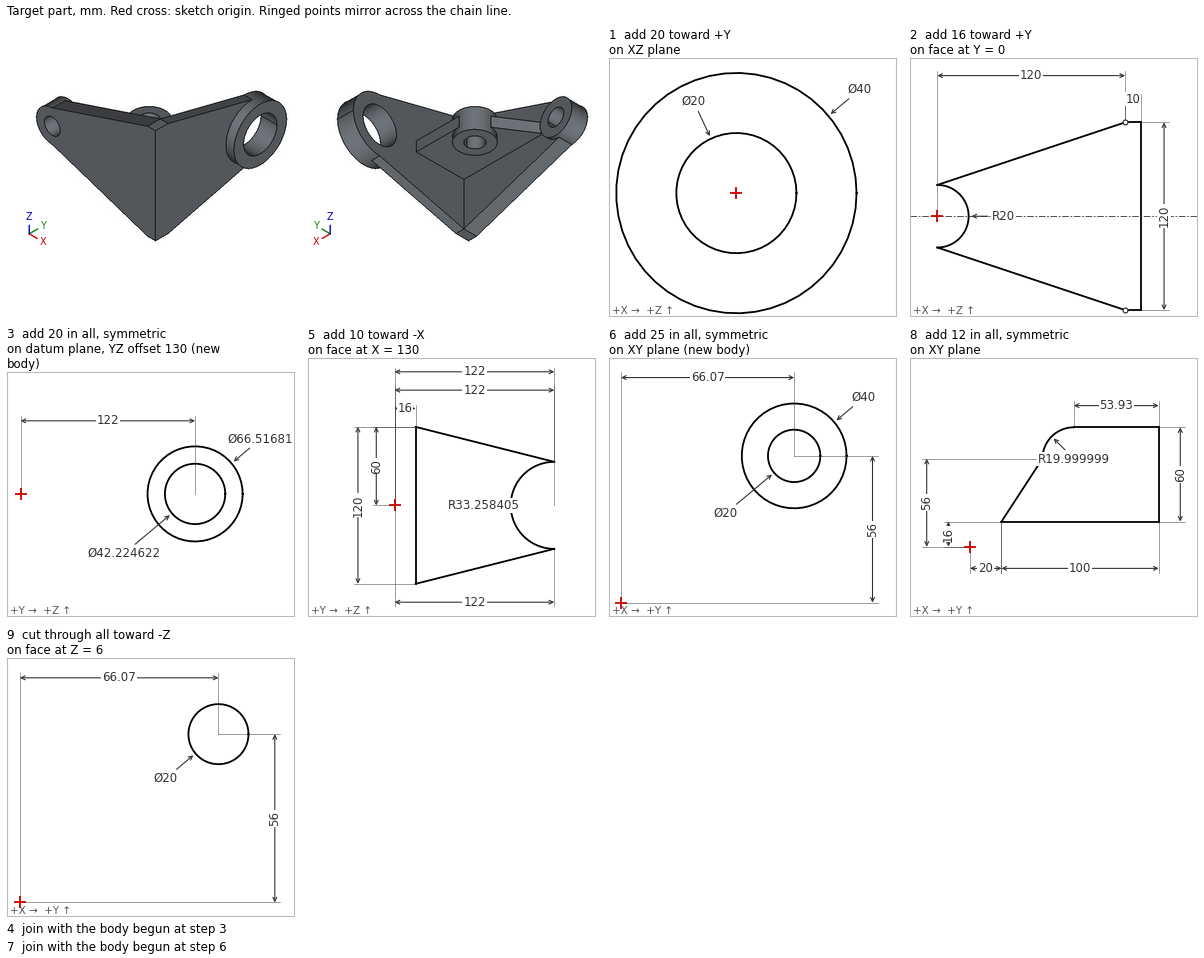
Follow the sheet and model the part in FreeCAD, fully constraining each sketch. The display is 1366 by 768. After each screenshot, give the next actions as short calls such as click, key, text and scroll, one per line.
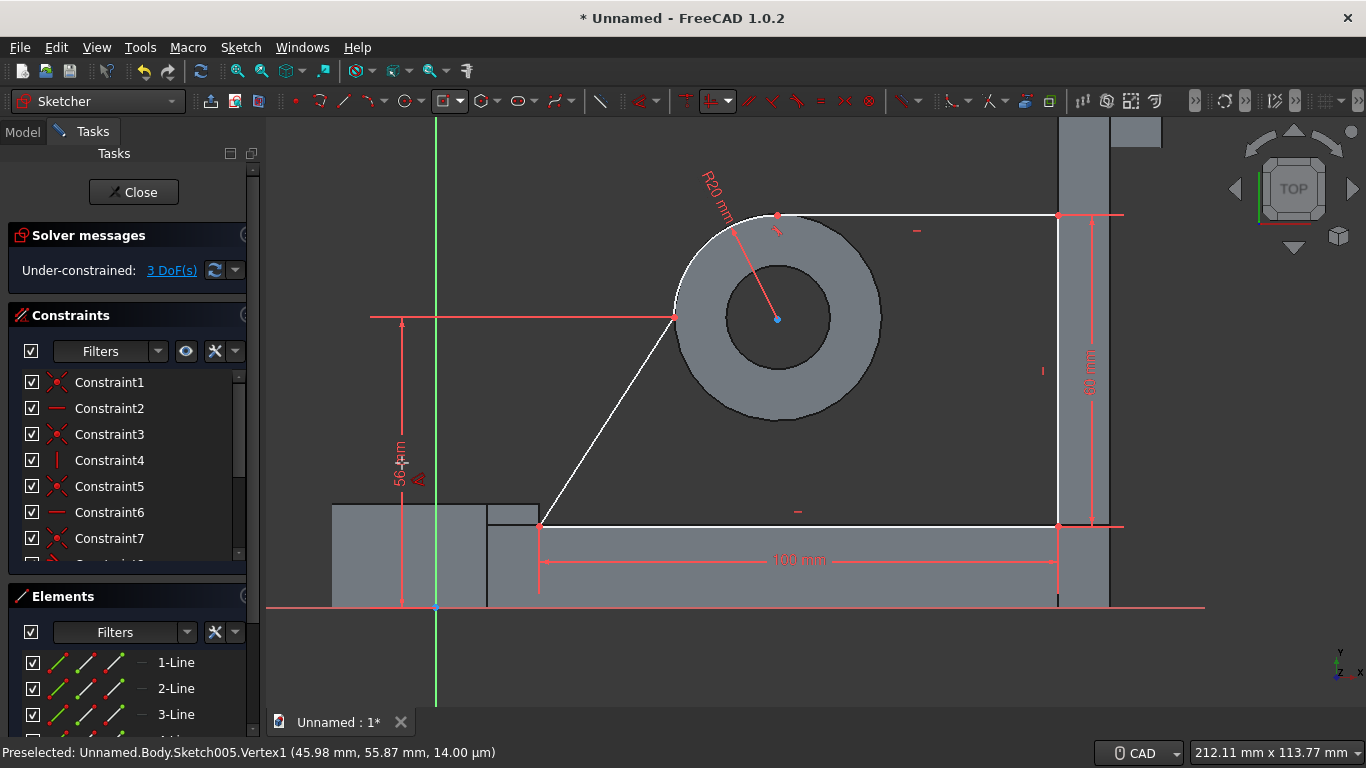
click(539, 527)
click(487, 642)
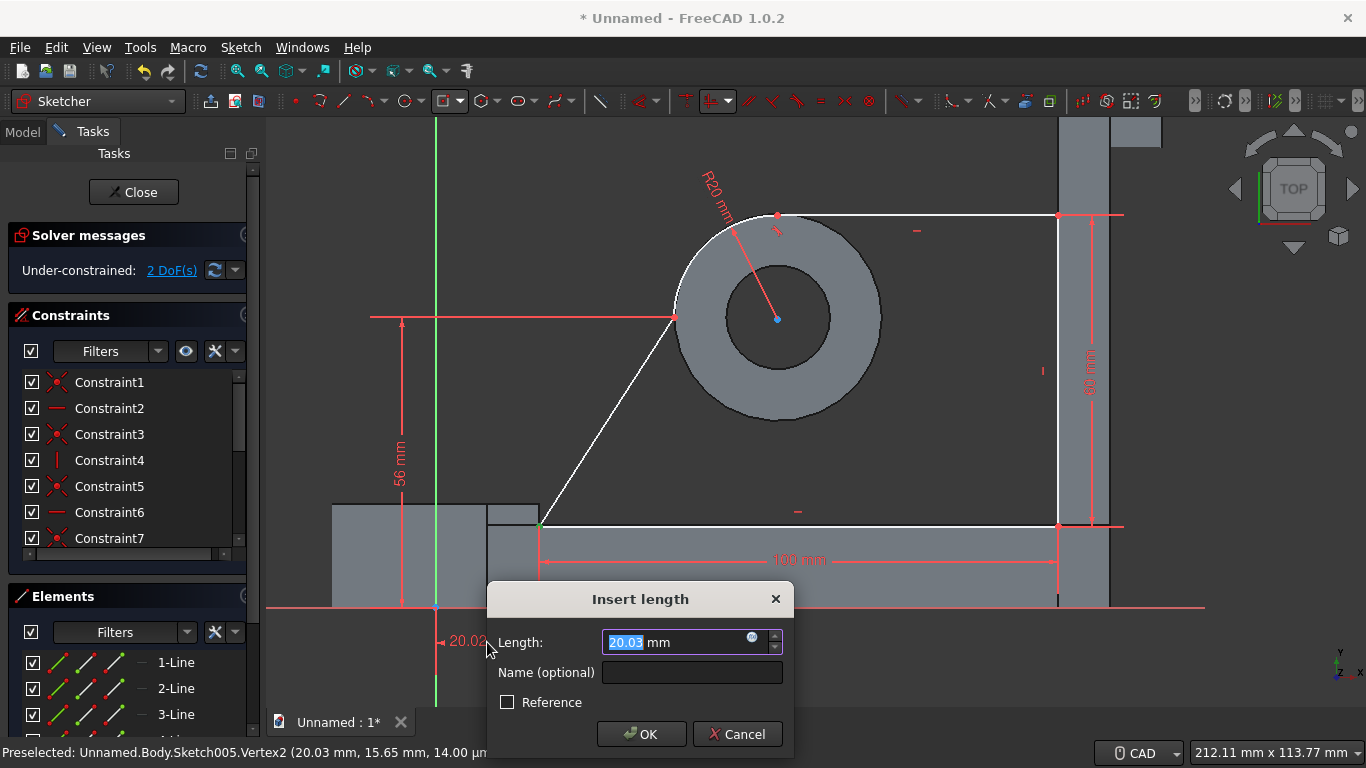
text(20)
key(Return)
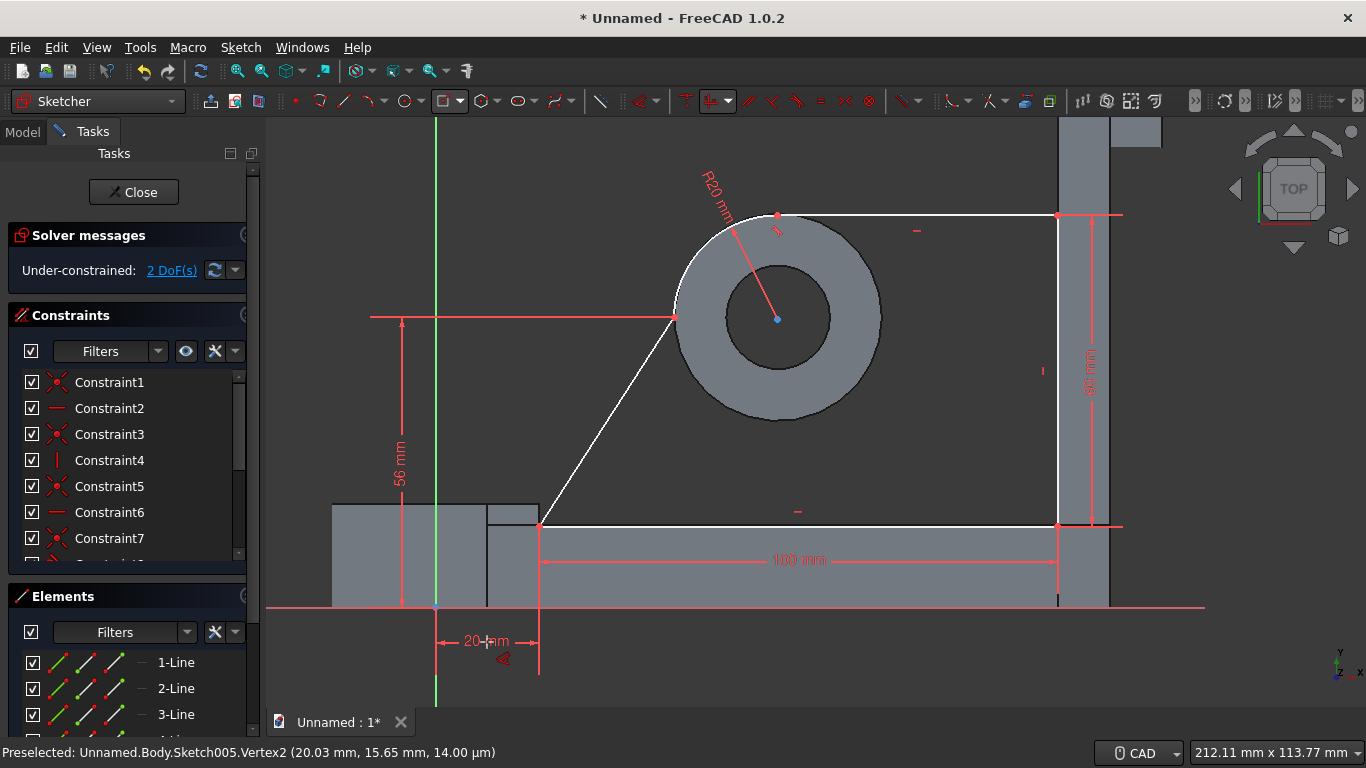
click(539, 527)
click(402, 567)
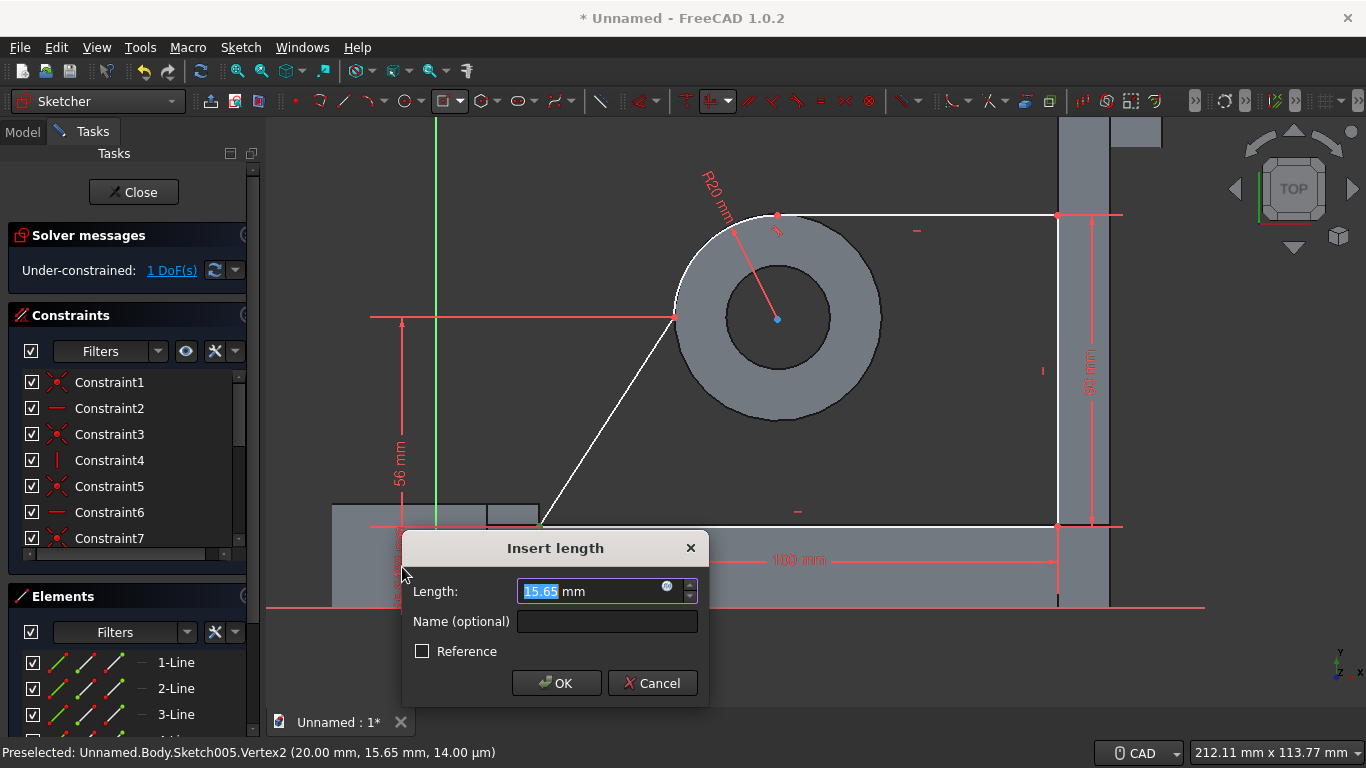
text(16)
key(Return)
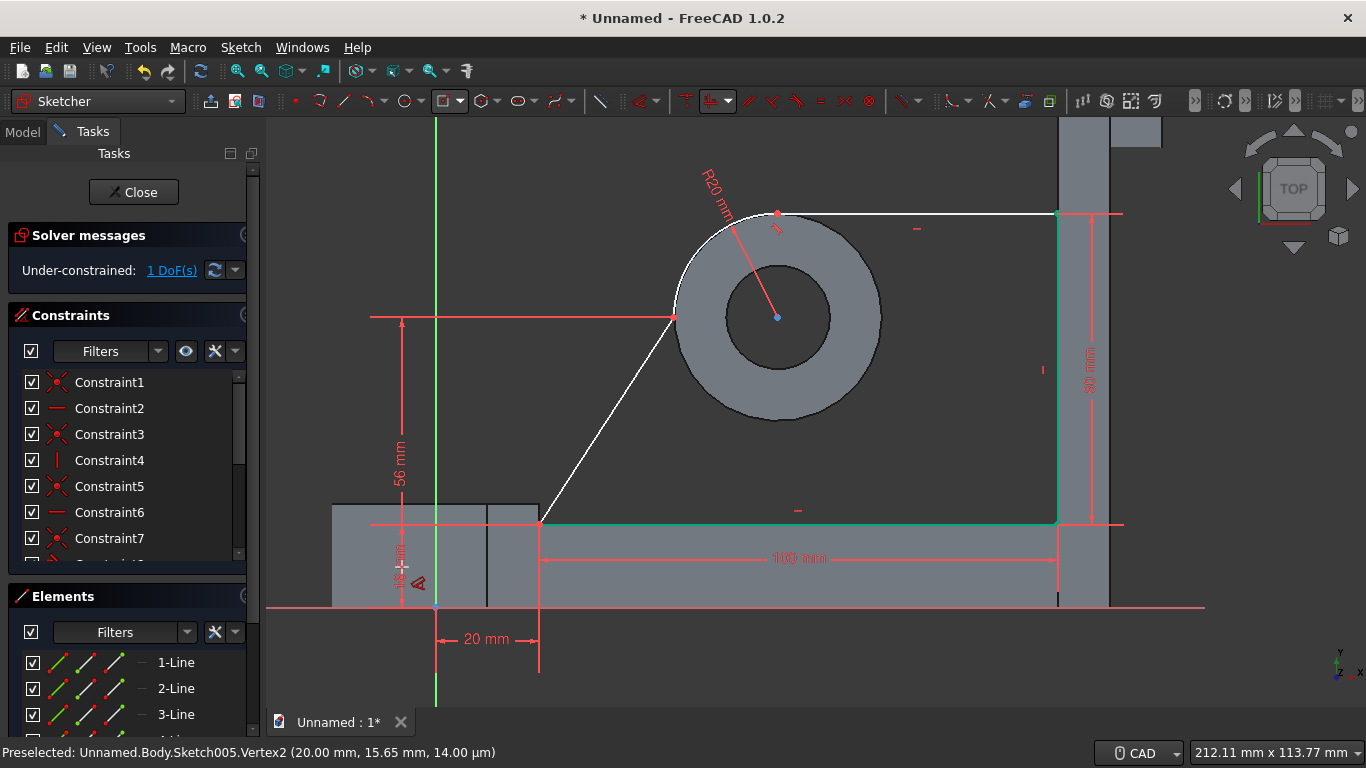
click(974, 214)
click(918, 180)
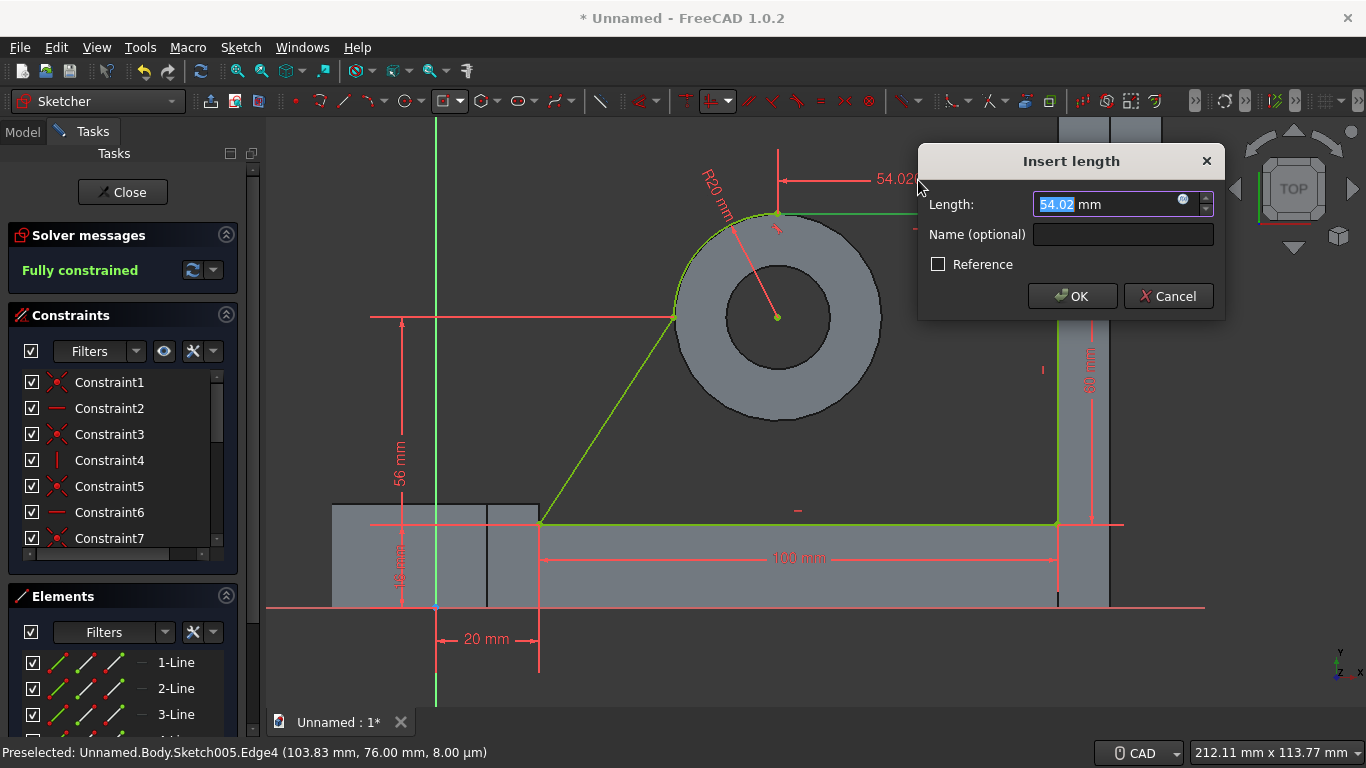
text(53.93)
key(Return)
key(Escape)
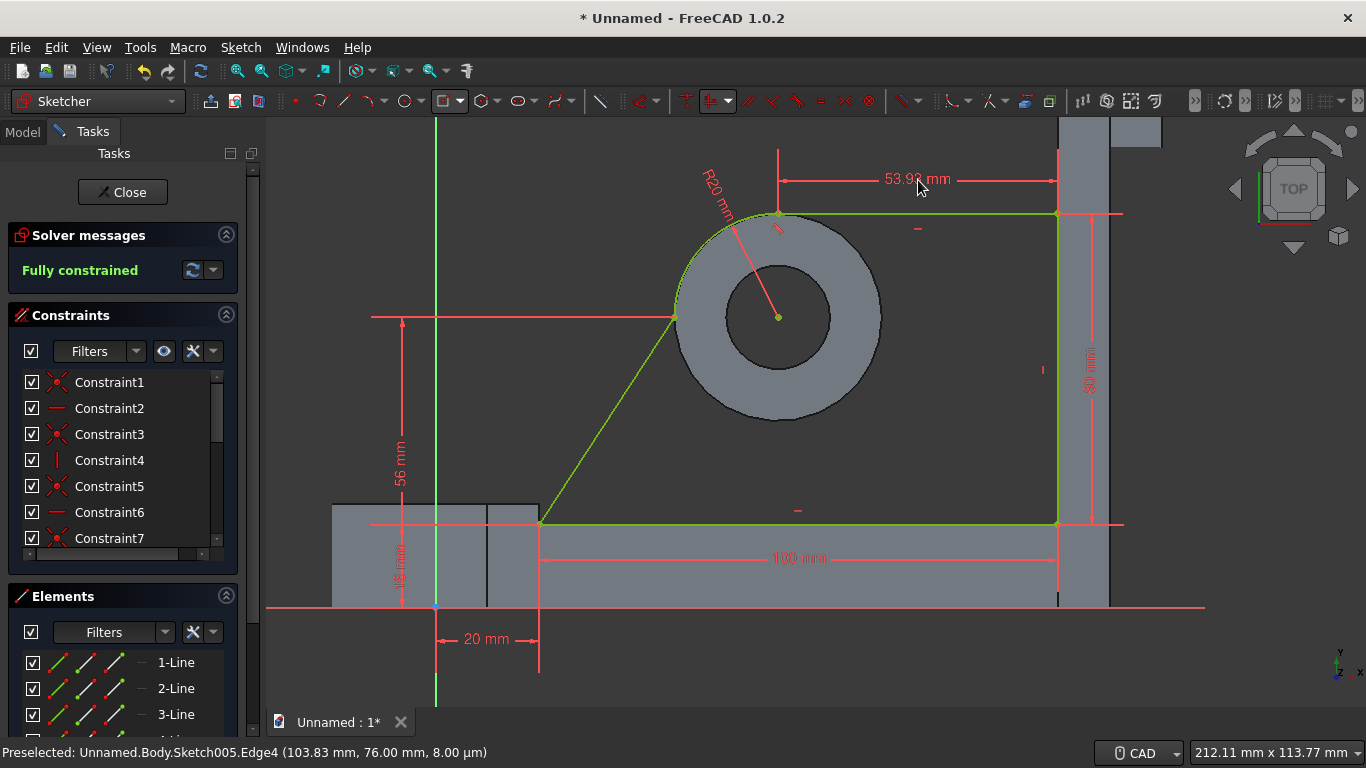
click(123, 192)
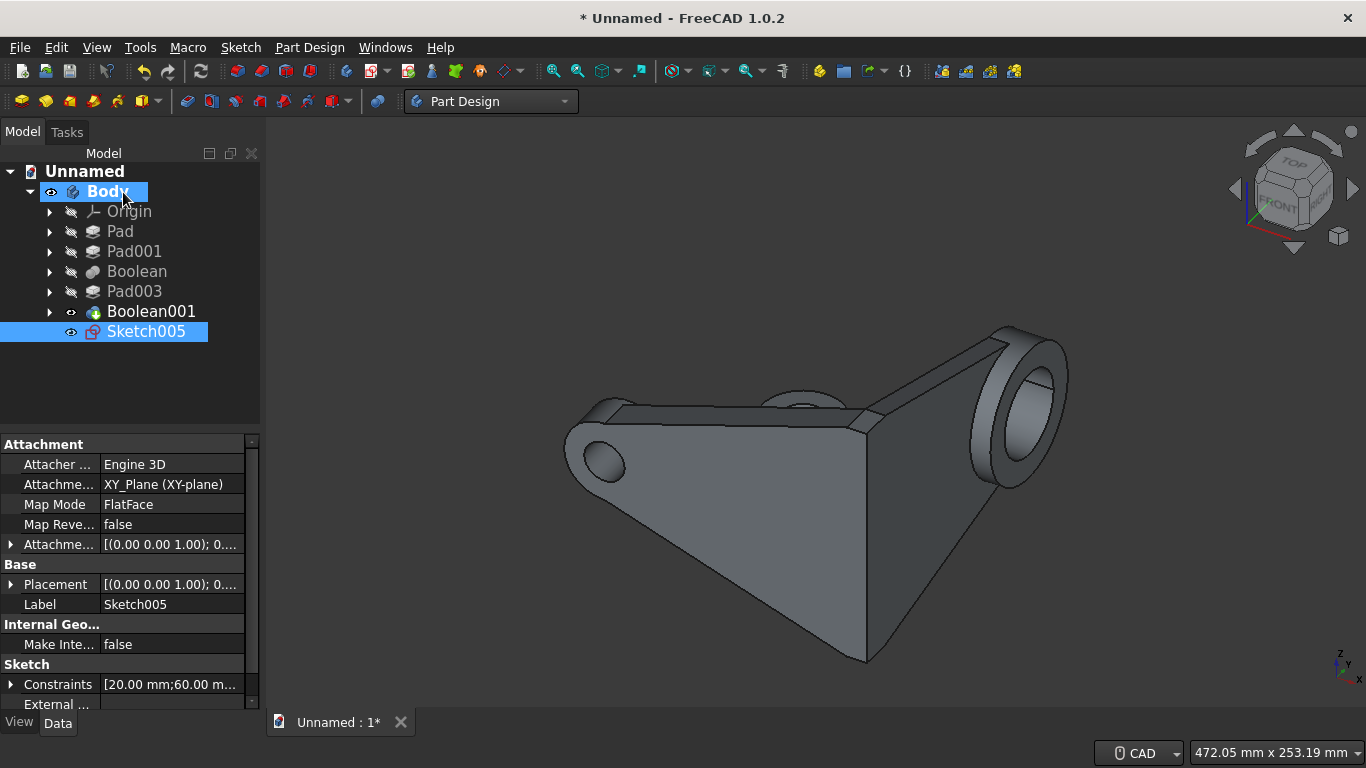
click(22, 102)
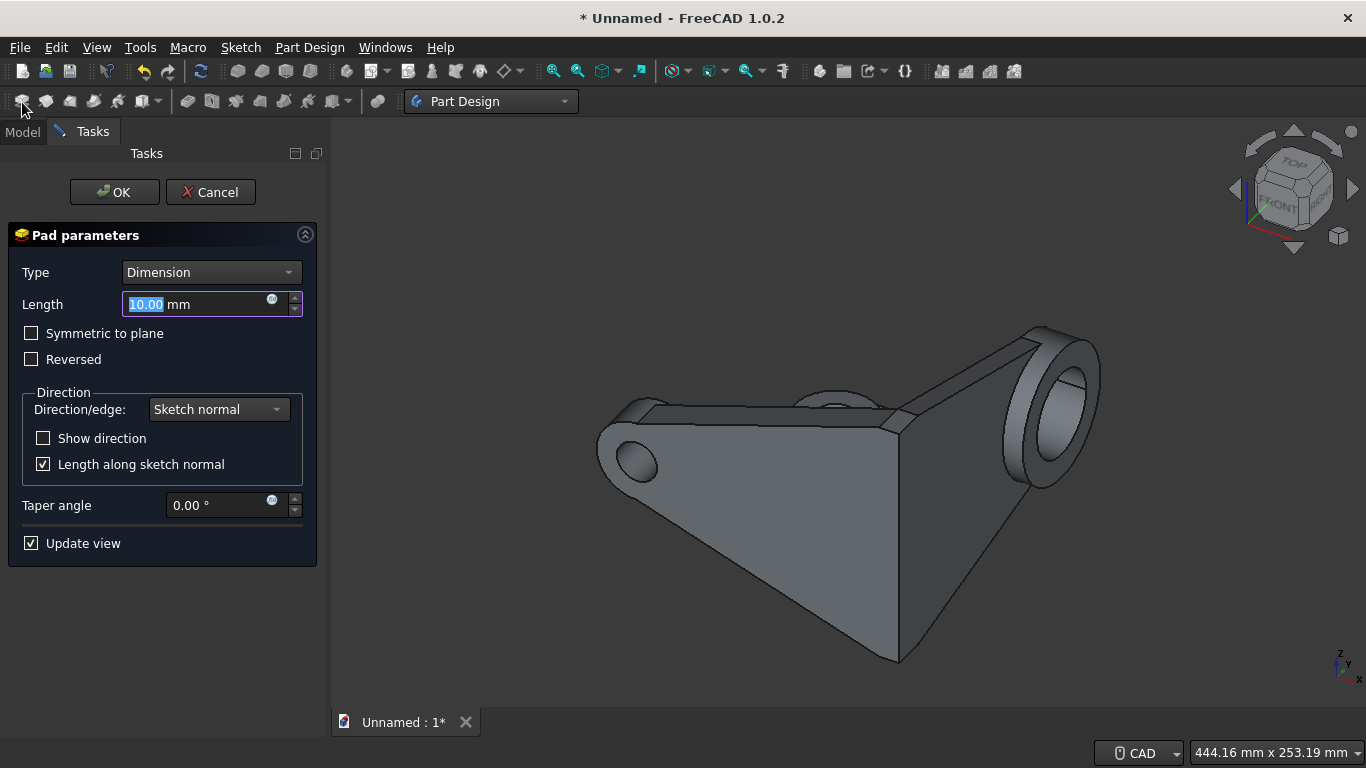
text(12)
key(Tab)